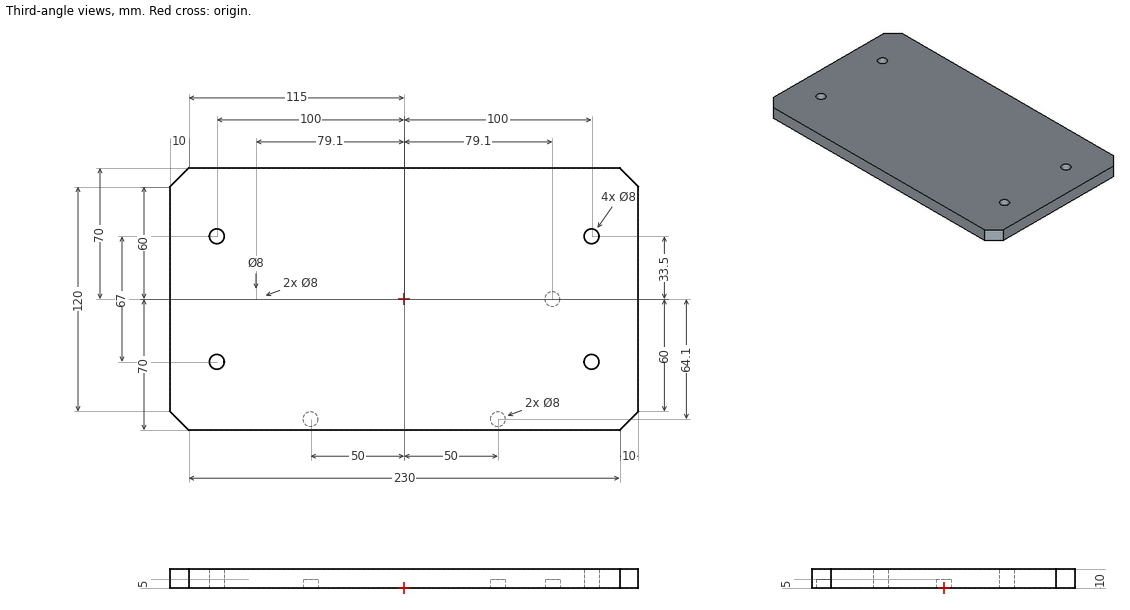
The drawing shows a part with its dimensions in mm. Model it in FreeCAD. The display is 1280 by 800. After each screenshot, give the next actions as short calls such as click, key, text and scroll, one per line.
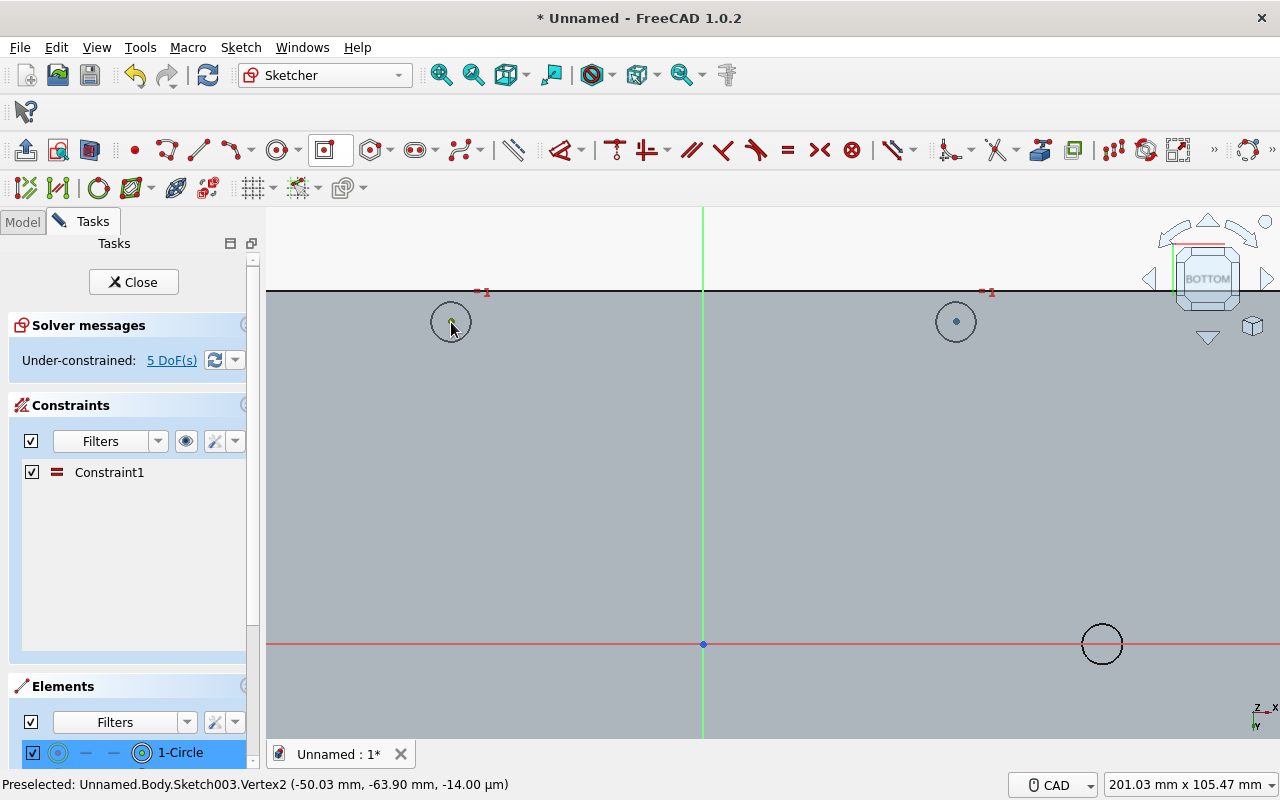
key(h)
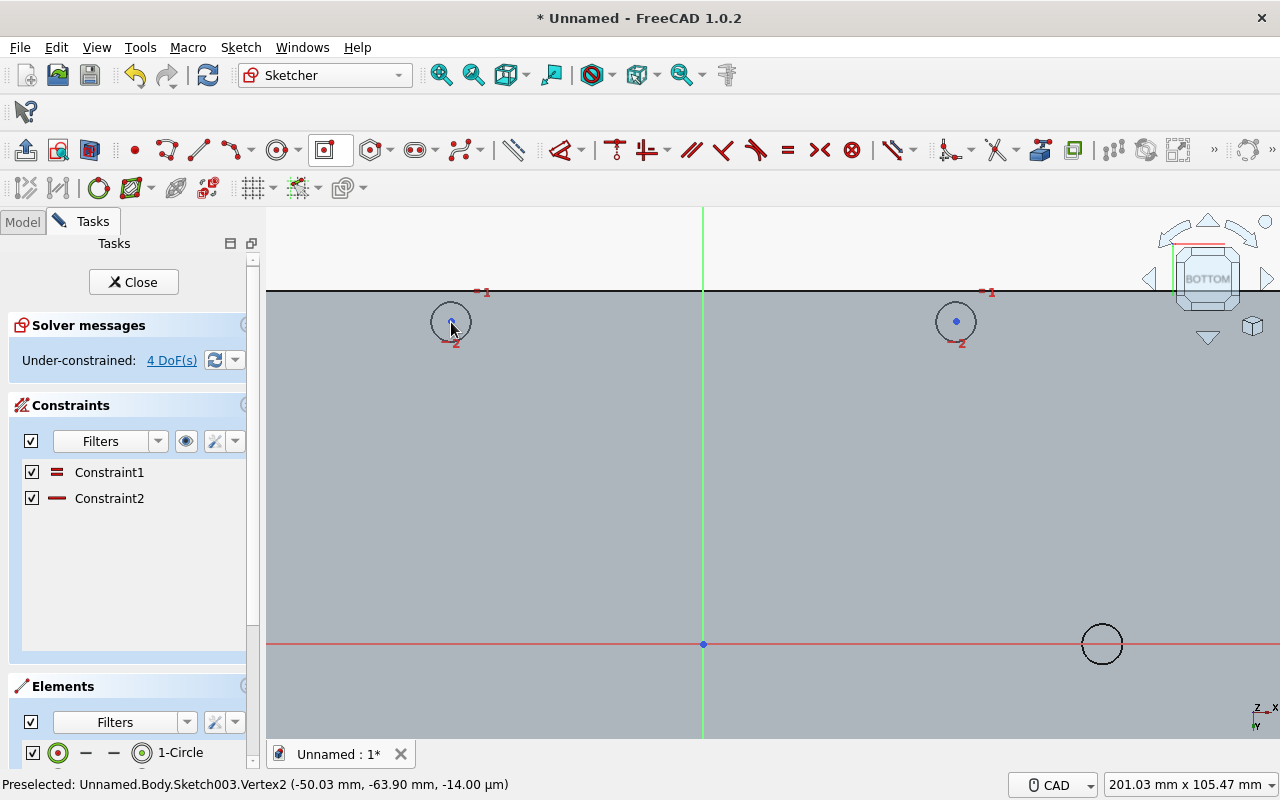
click(560, 150)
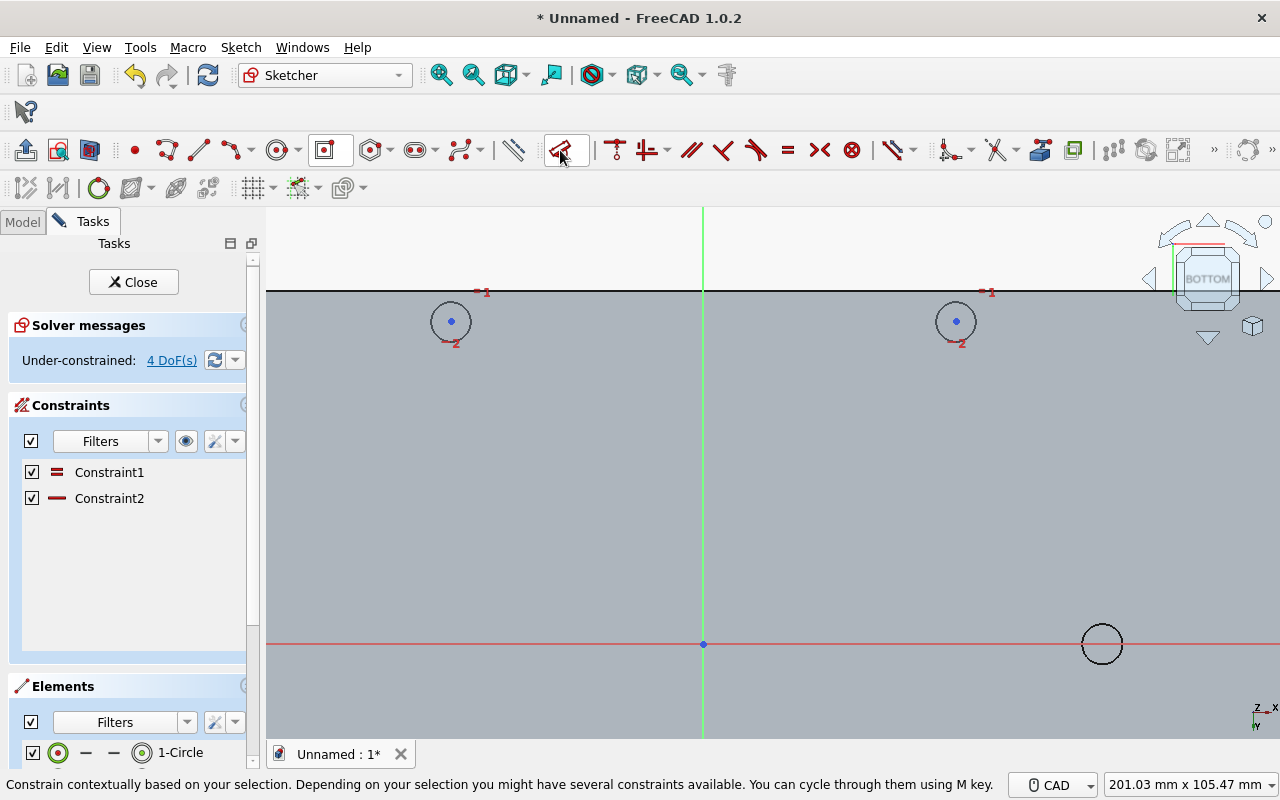
click(970, 308)
click(993, 285)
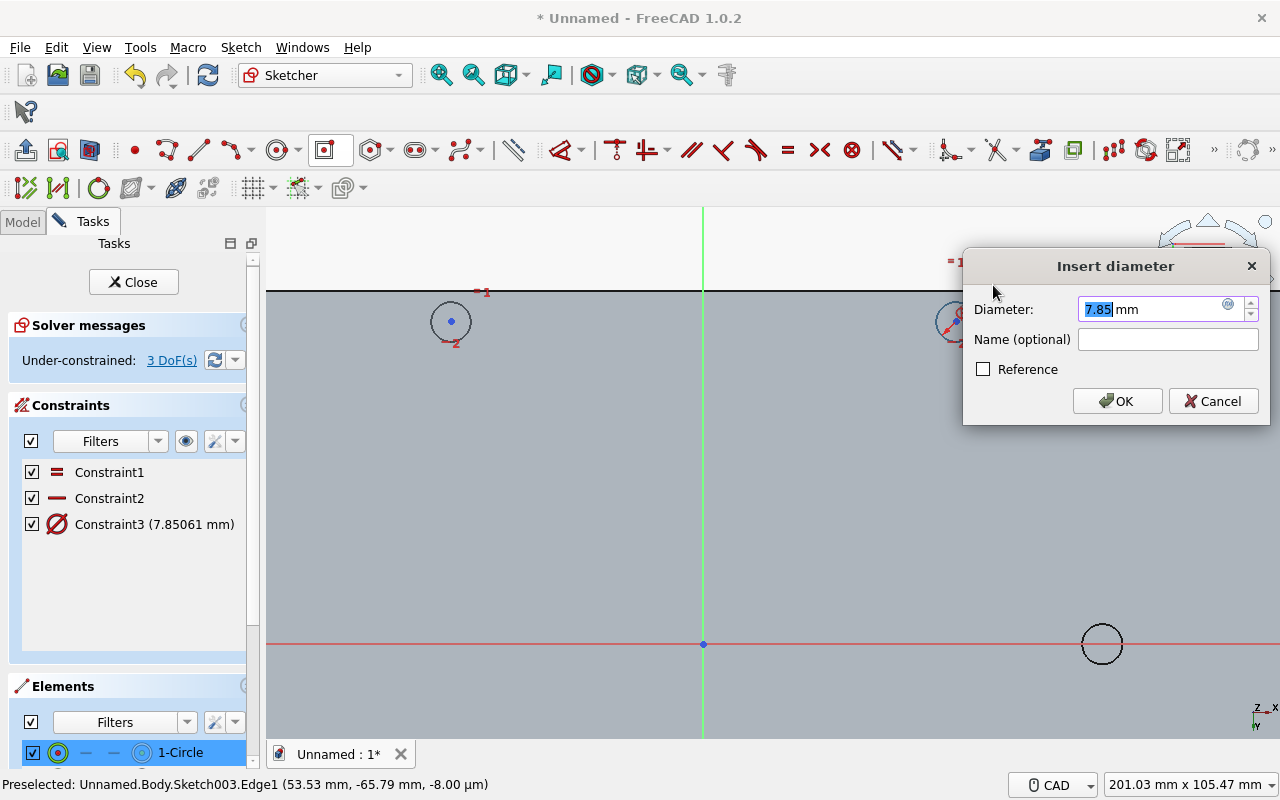
text(8)
key(Return)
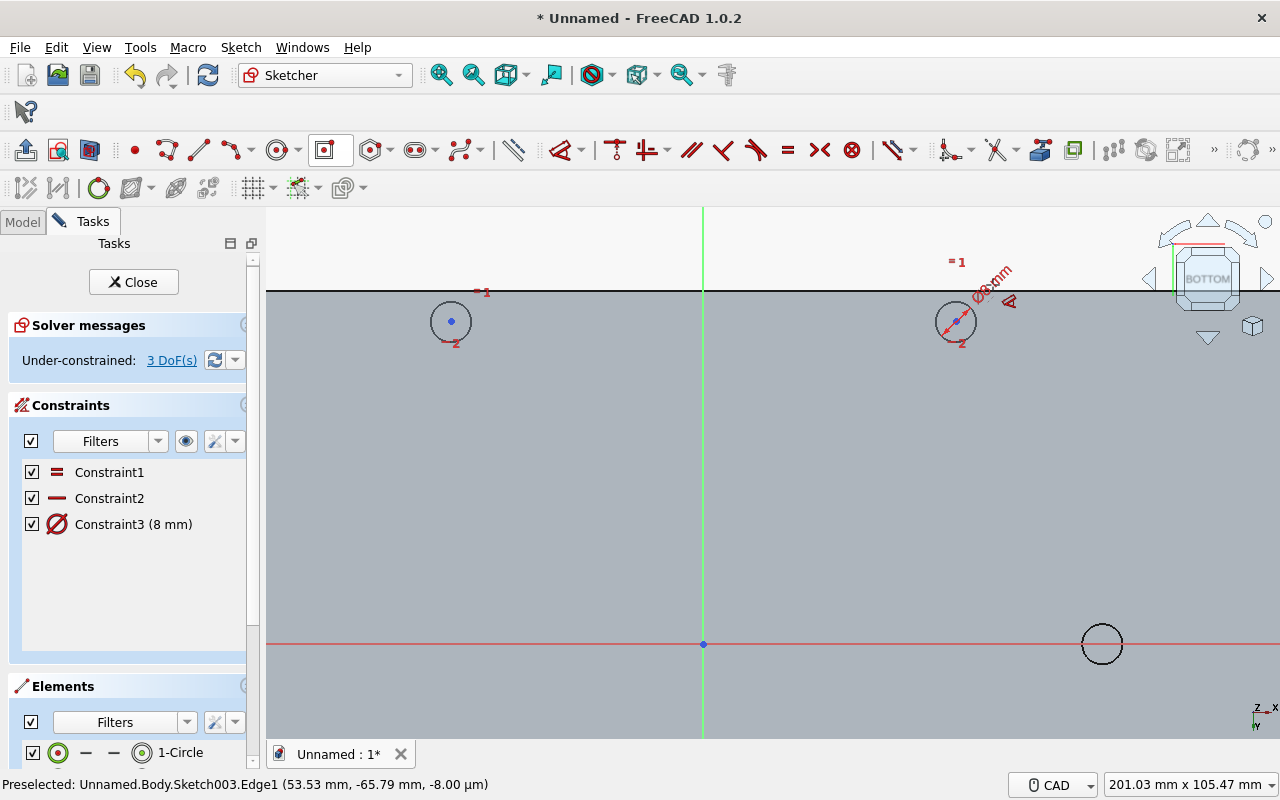
click(956, 322)
click(830, 678)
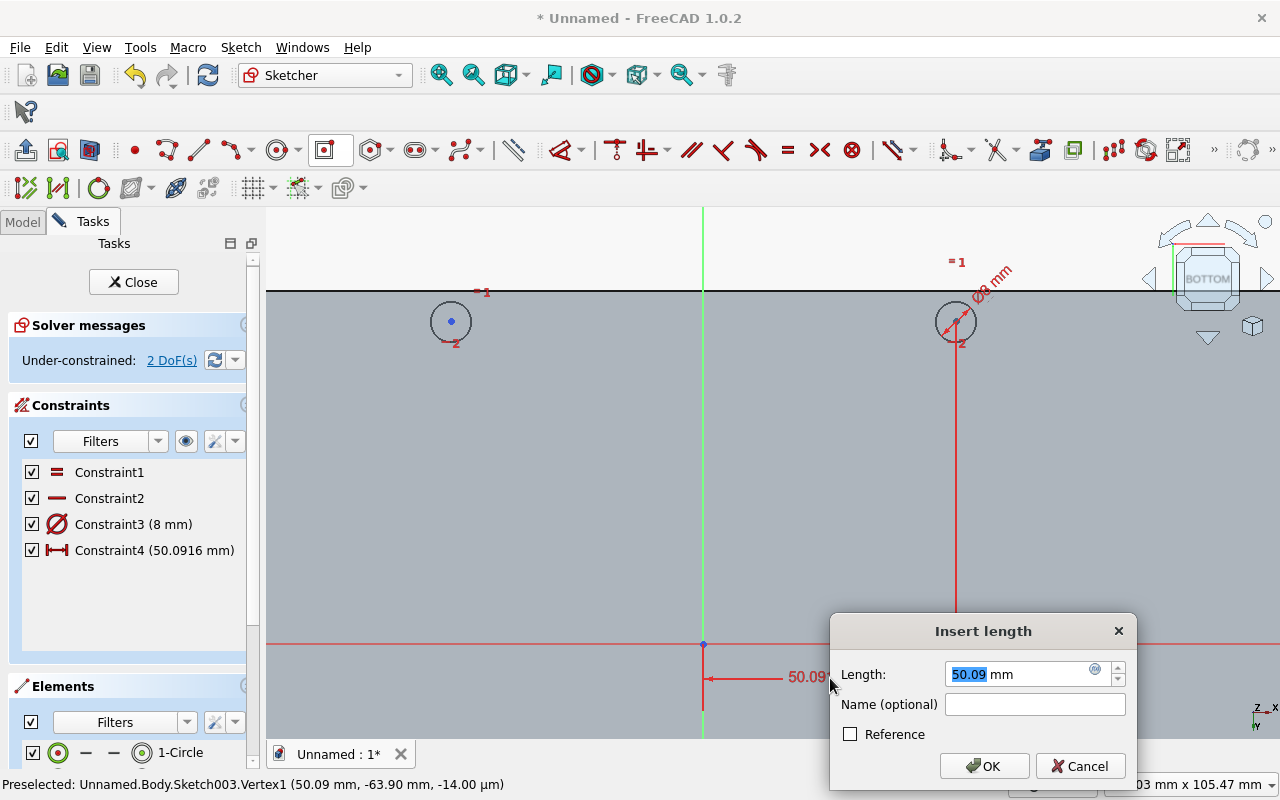
text(50)
key(Return)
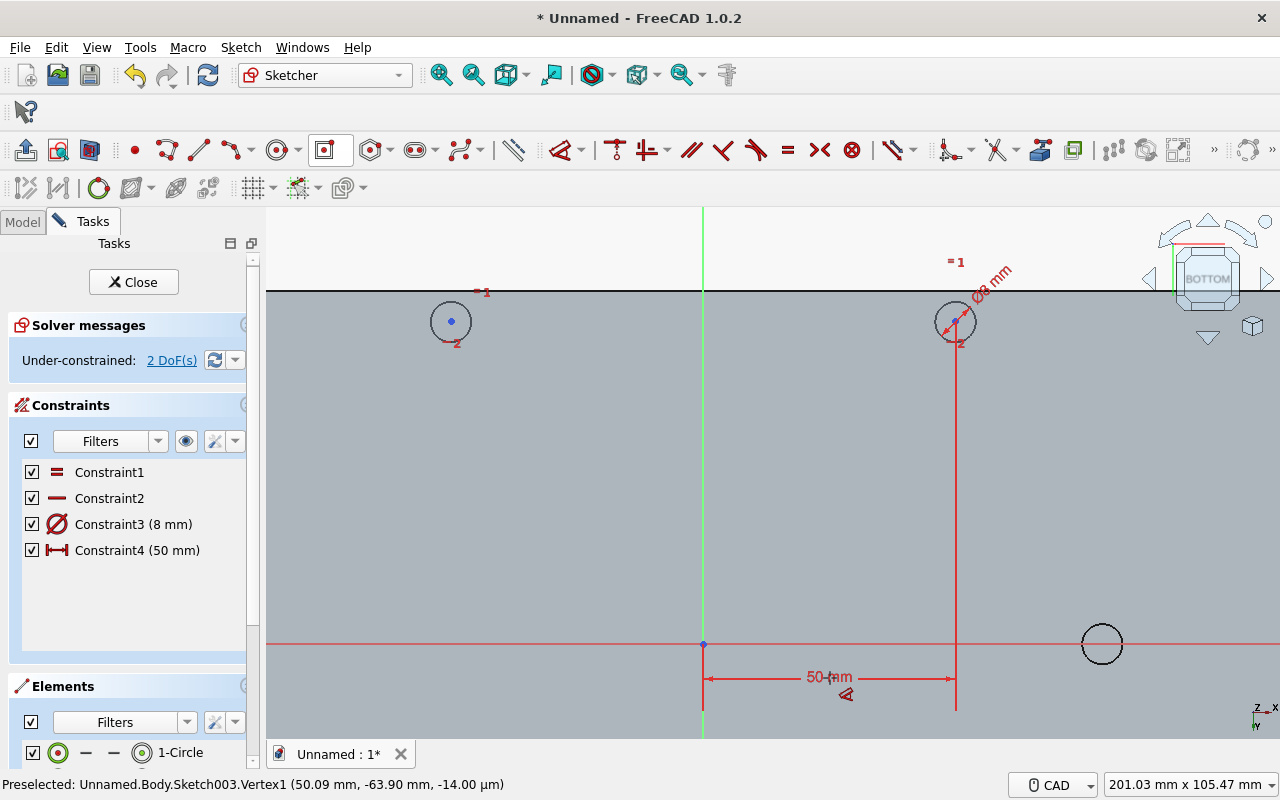
click(451, 322)
click(577, 678)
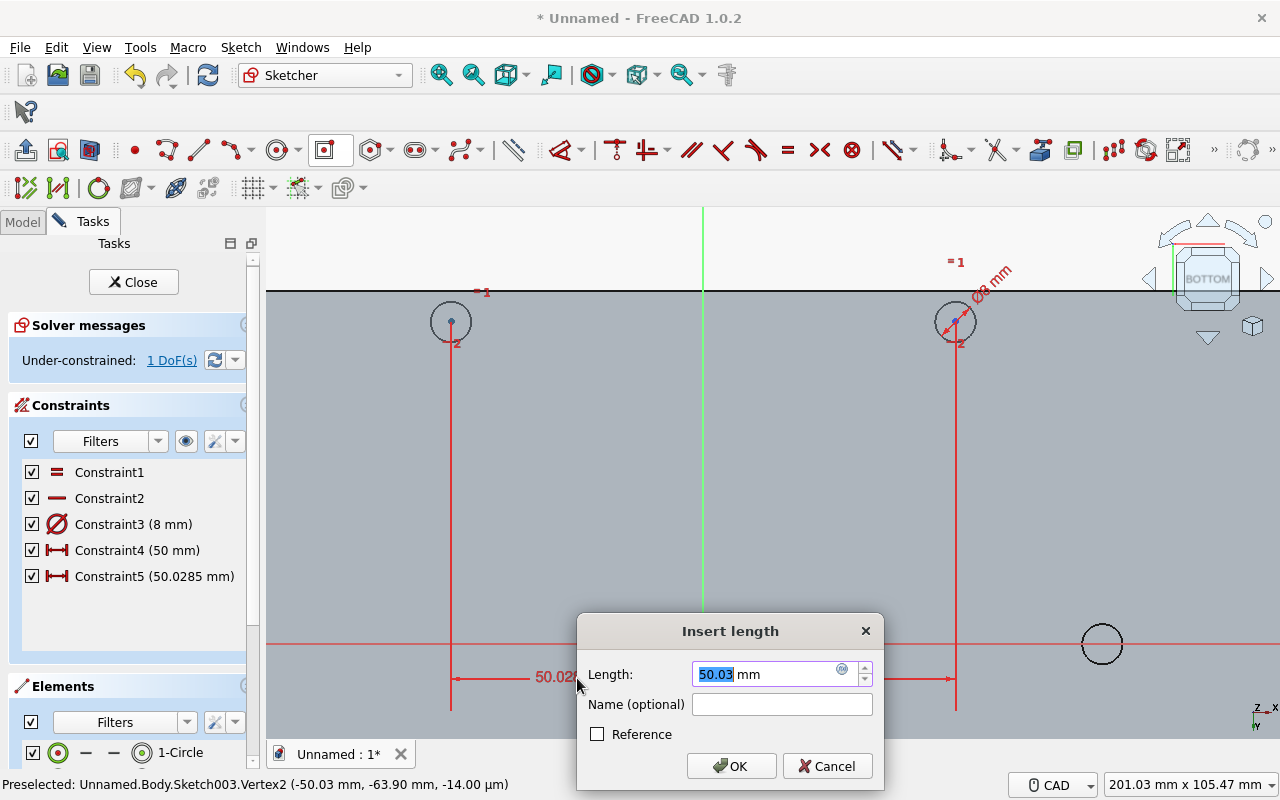
text(50)
key(Return)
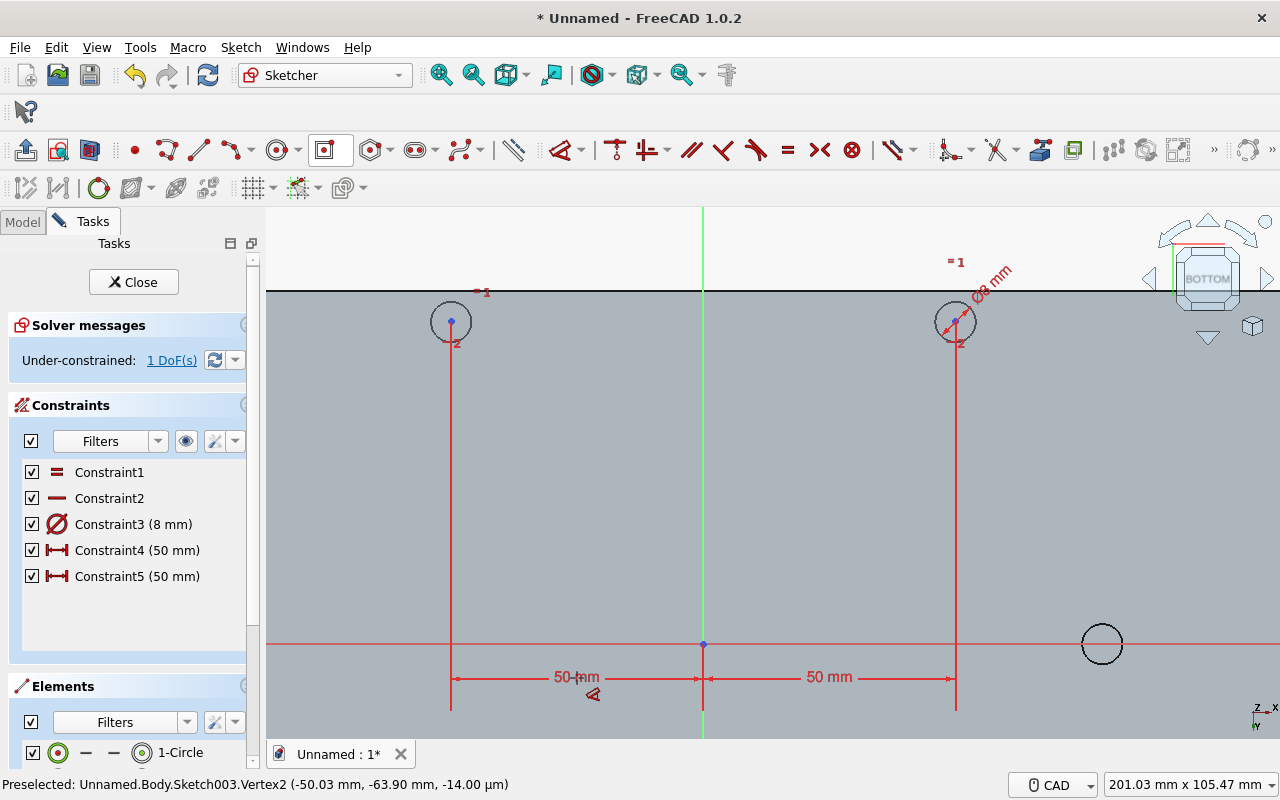
click(956, 322)
click(990, 483)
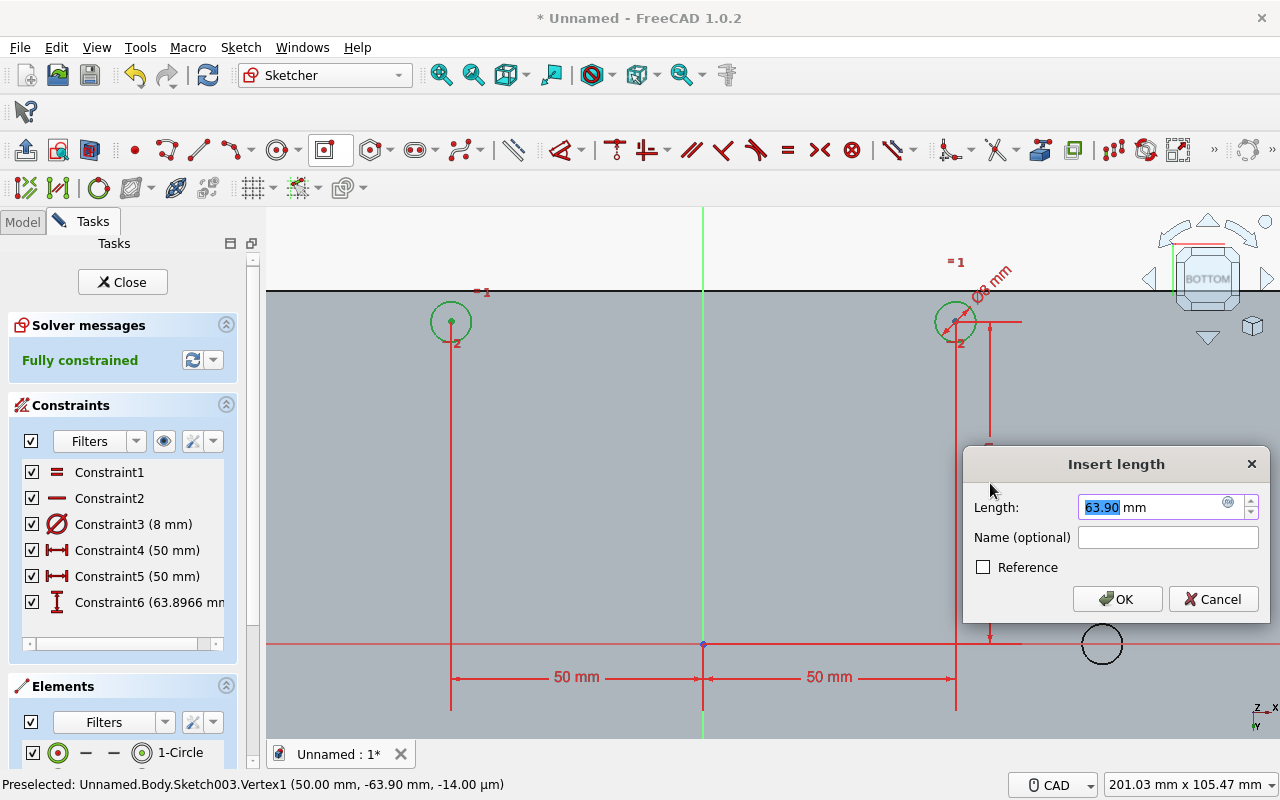
text(64.1)
key(Return)
key(Escape)